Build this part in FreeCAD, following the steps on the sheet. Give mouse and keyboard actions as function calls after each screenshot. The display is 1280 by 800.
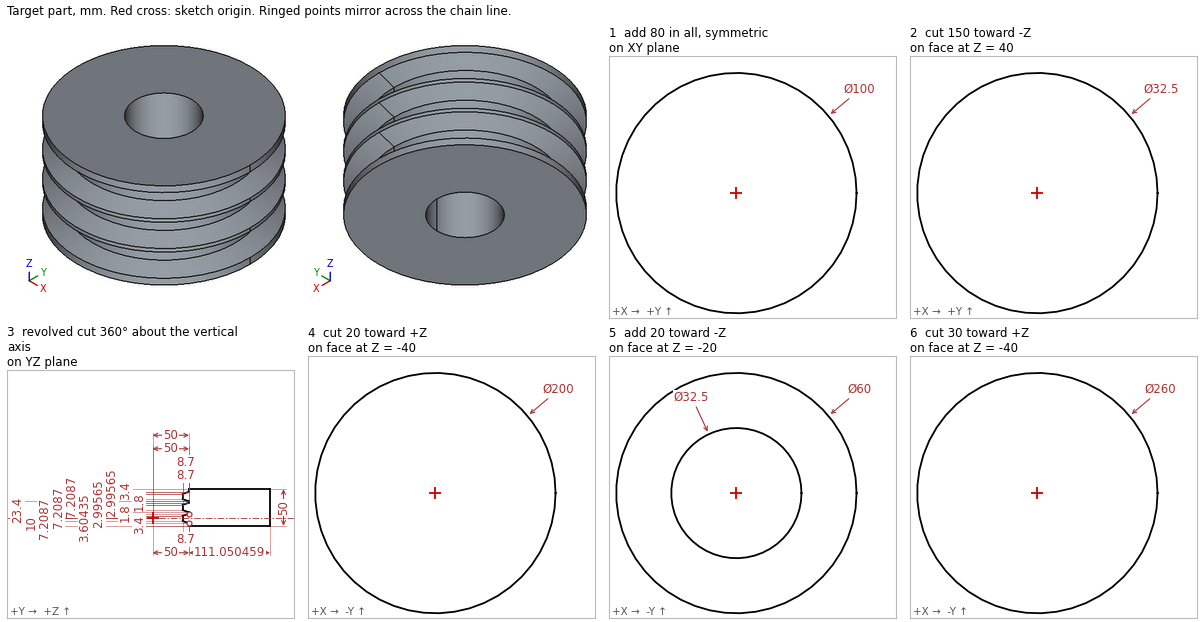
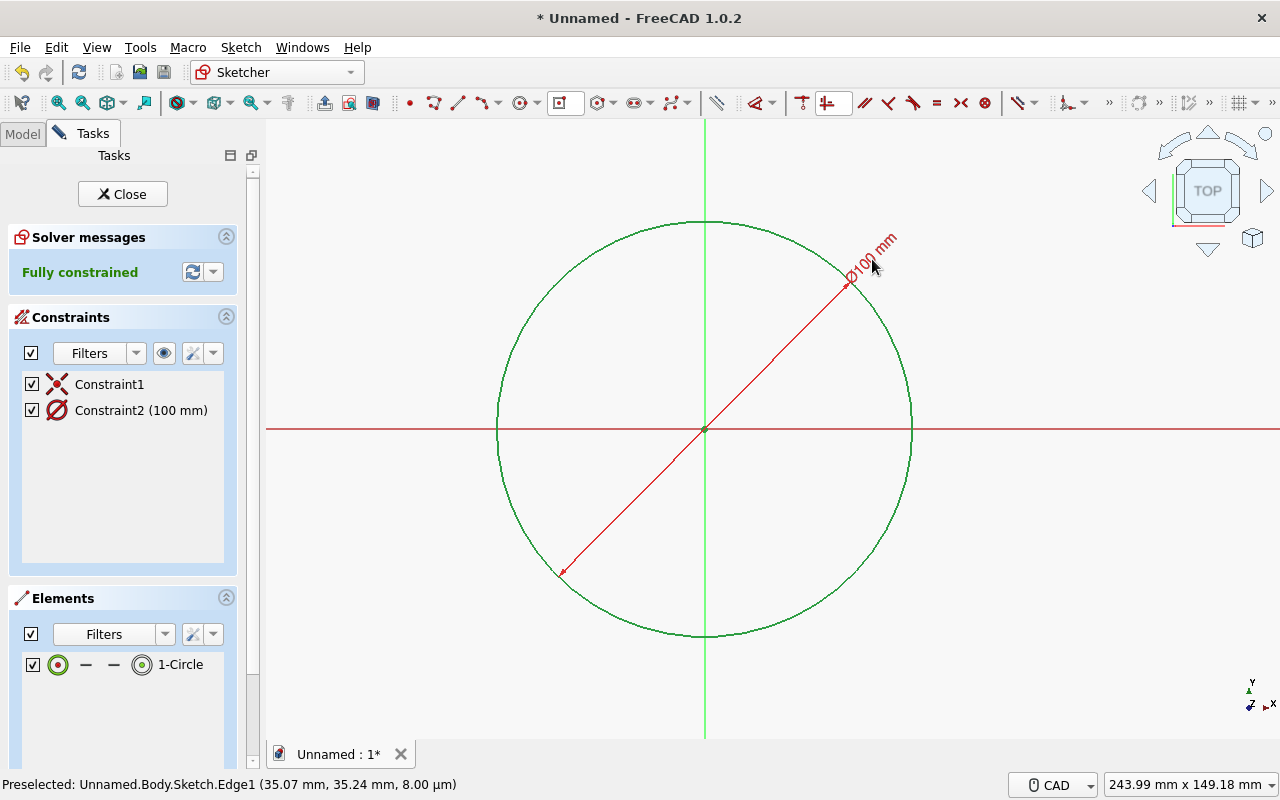
click(123, 194)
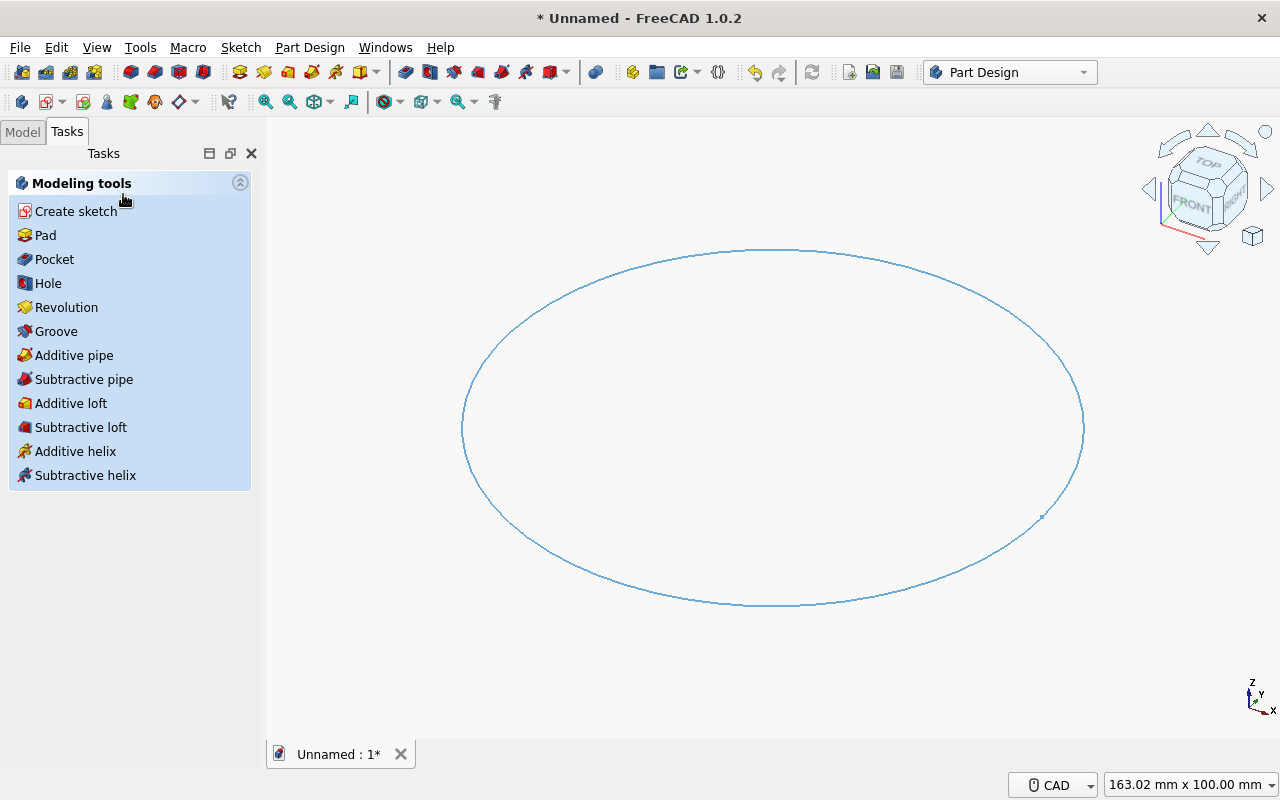
click(240, 72)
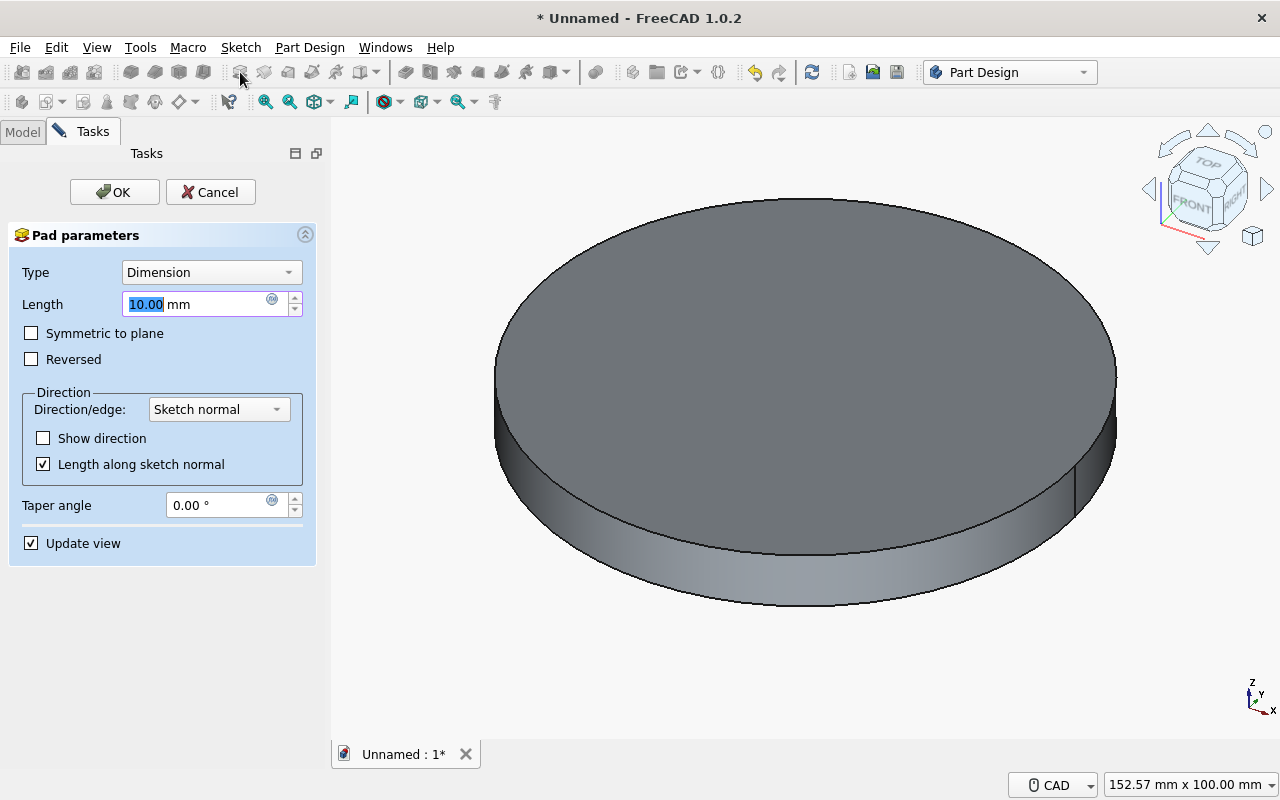
text(80)
key(Tab)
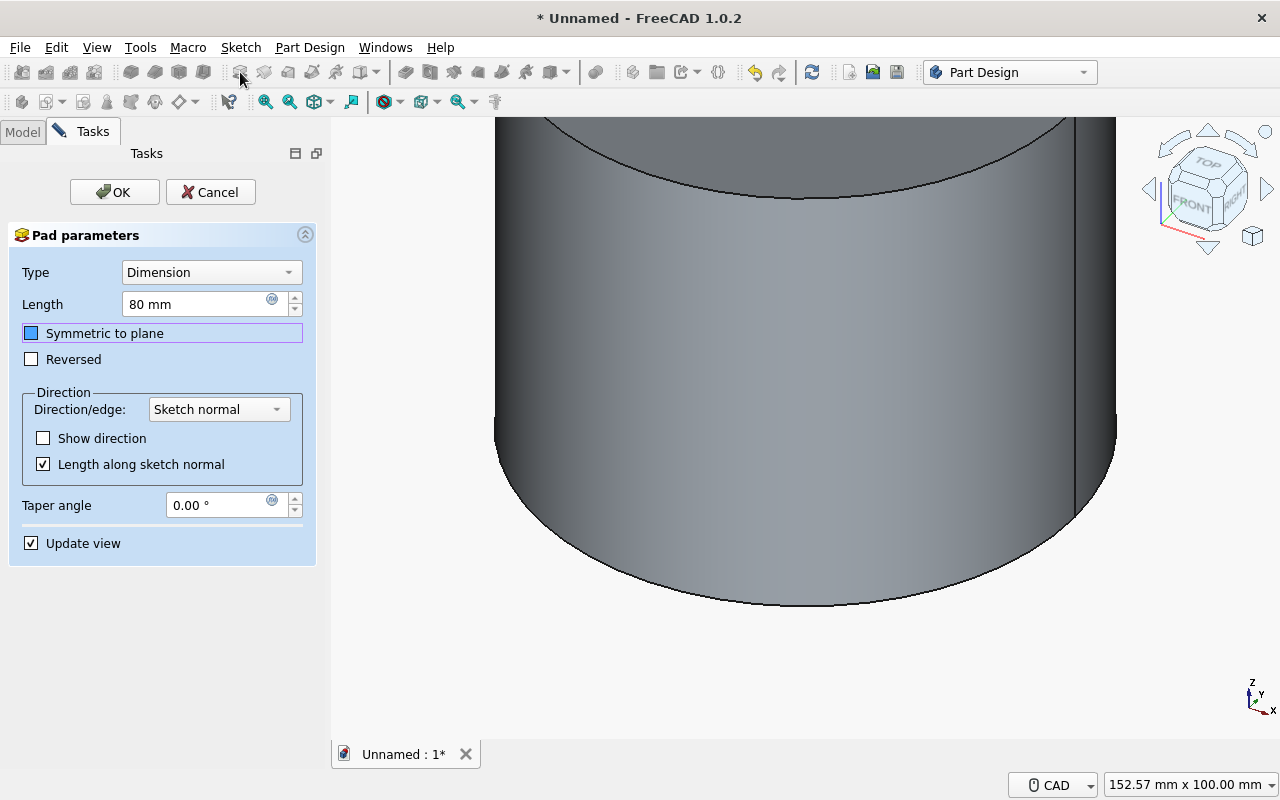
click(30, 333)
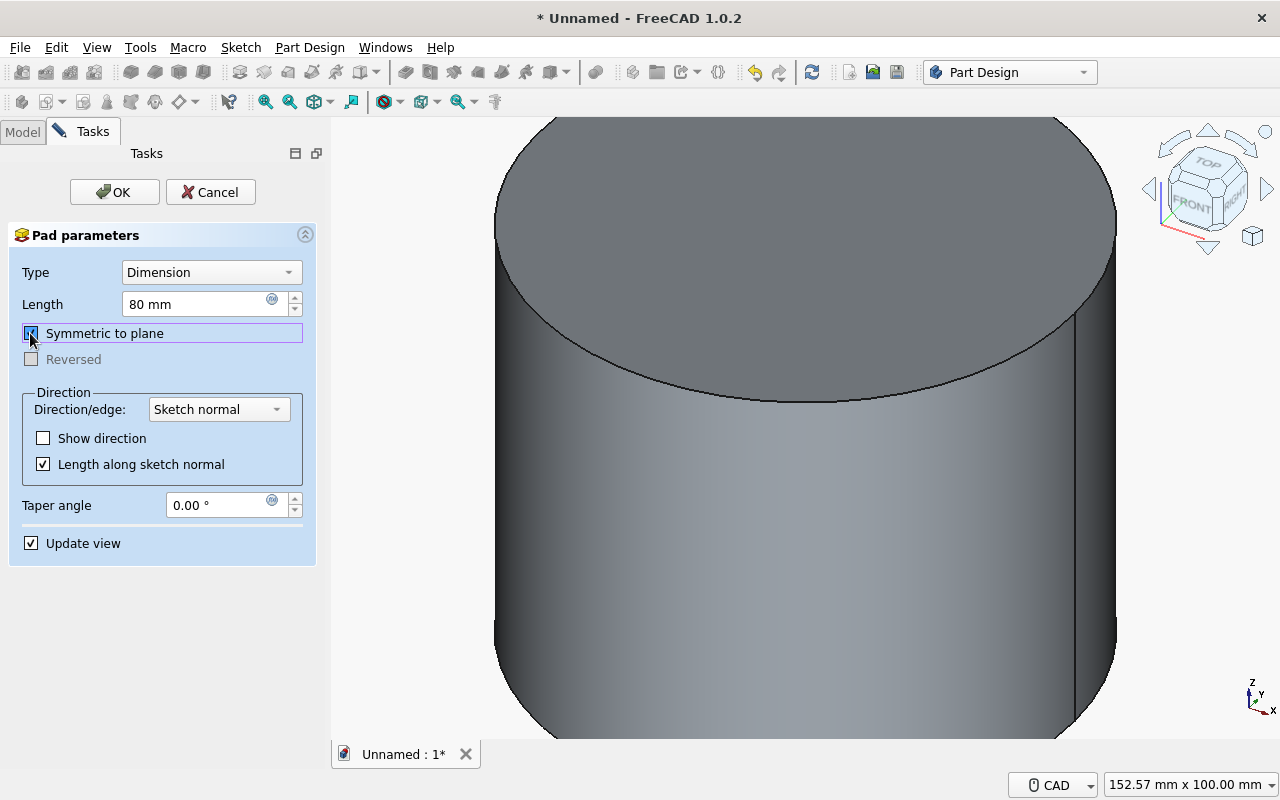
click(115, 192)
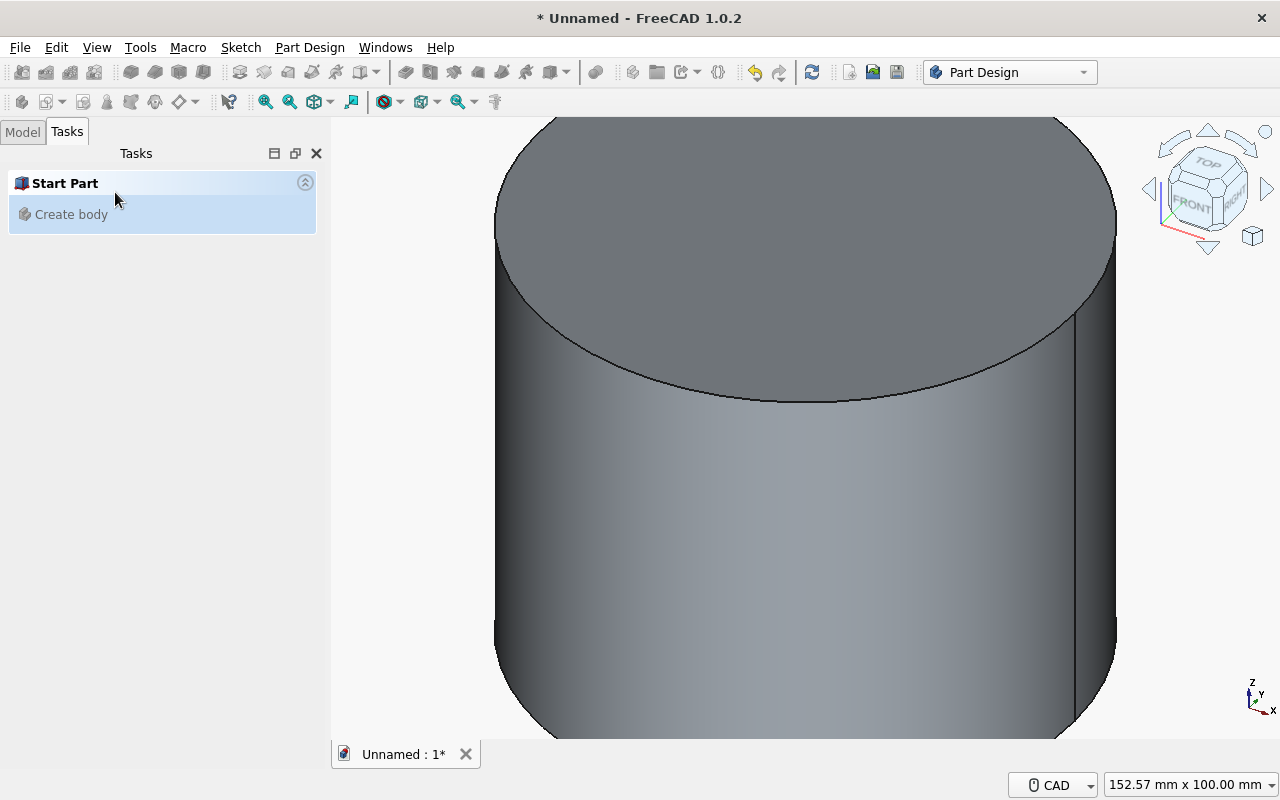
click(266, 102)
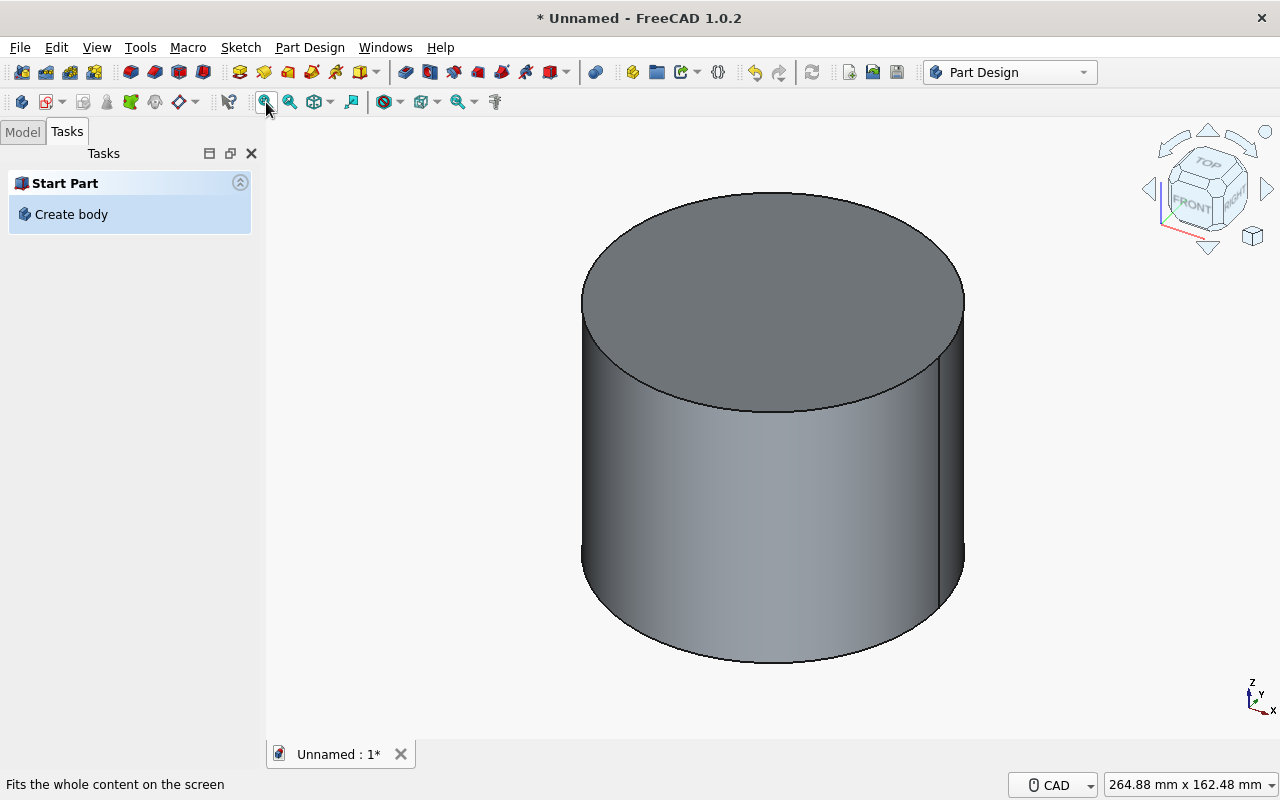
click(773, 302)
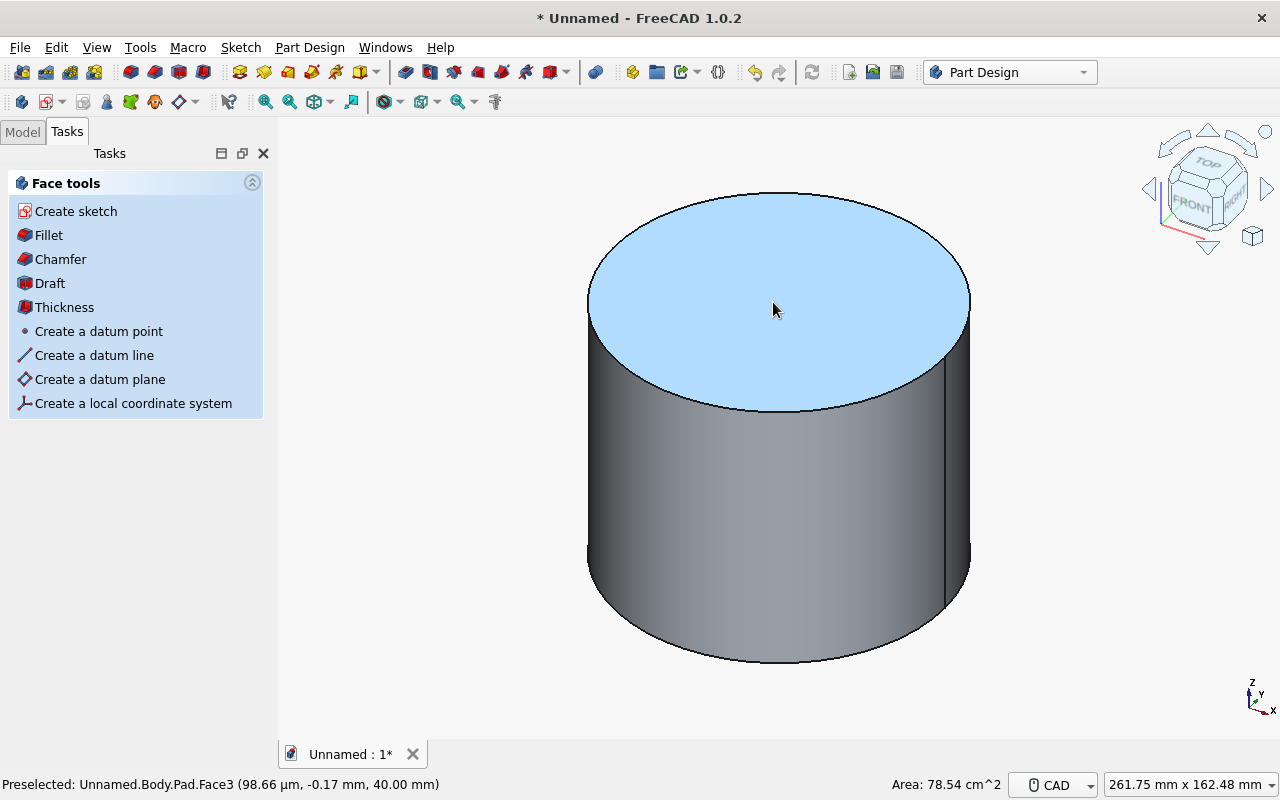
click(46, 102)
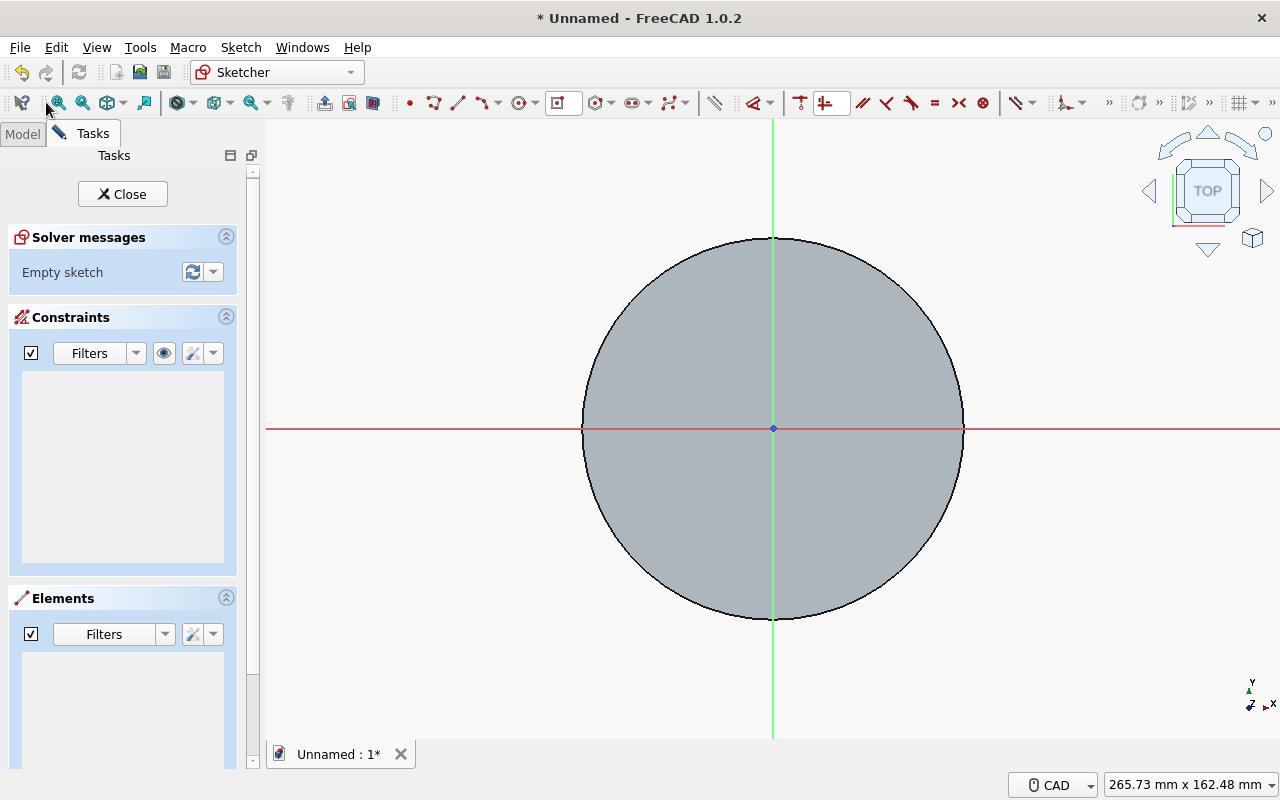
scroll(803, 429, up, 6)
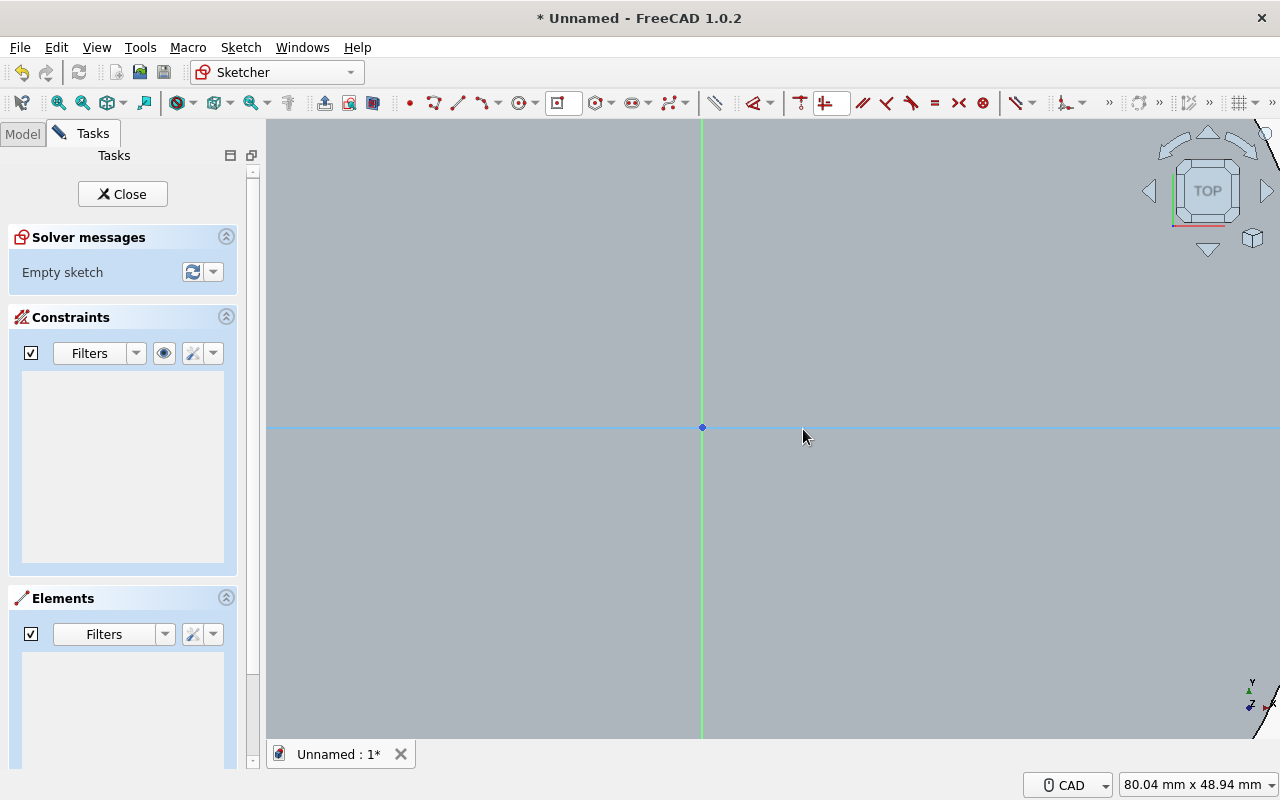
click(520, 104)